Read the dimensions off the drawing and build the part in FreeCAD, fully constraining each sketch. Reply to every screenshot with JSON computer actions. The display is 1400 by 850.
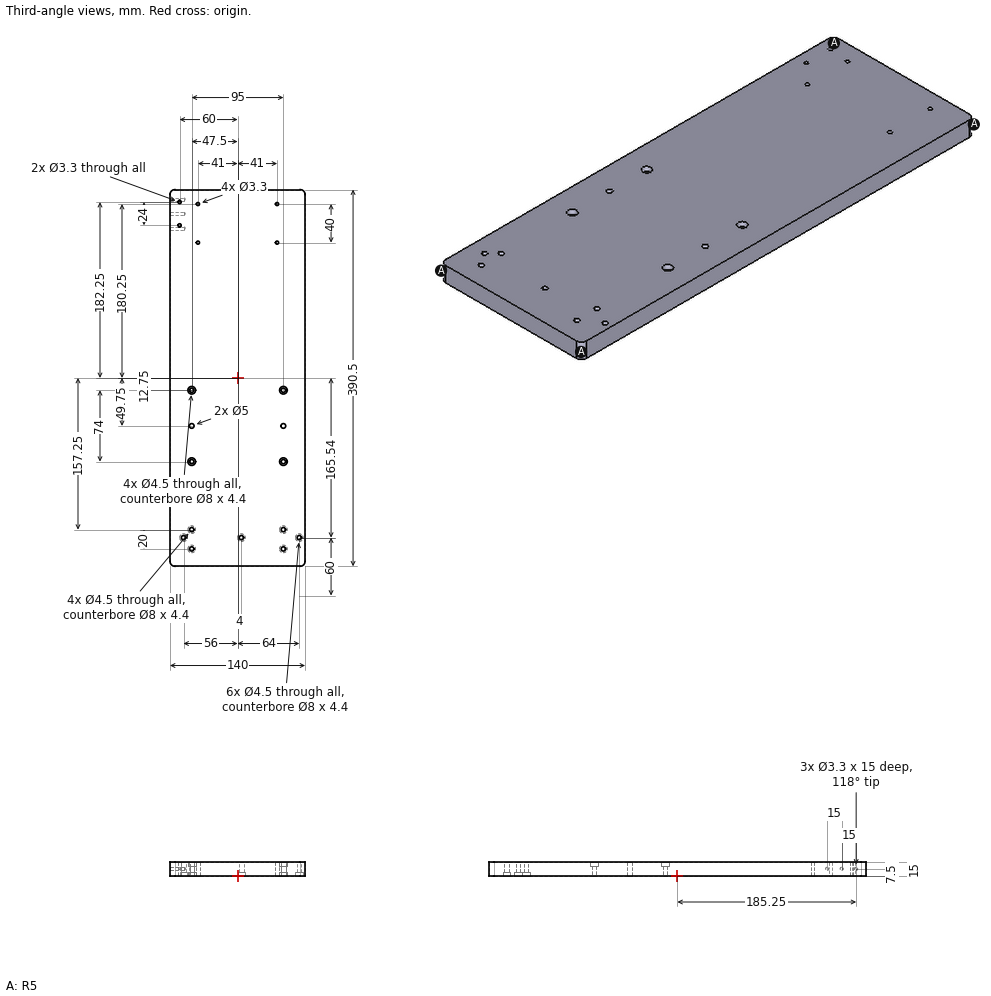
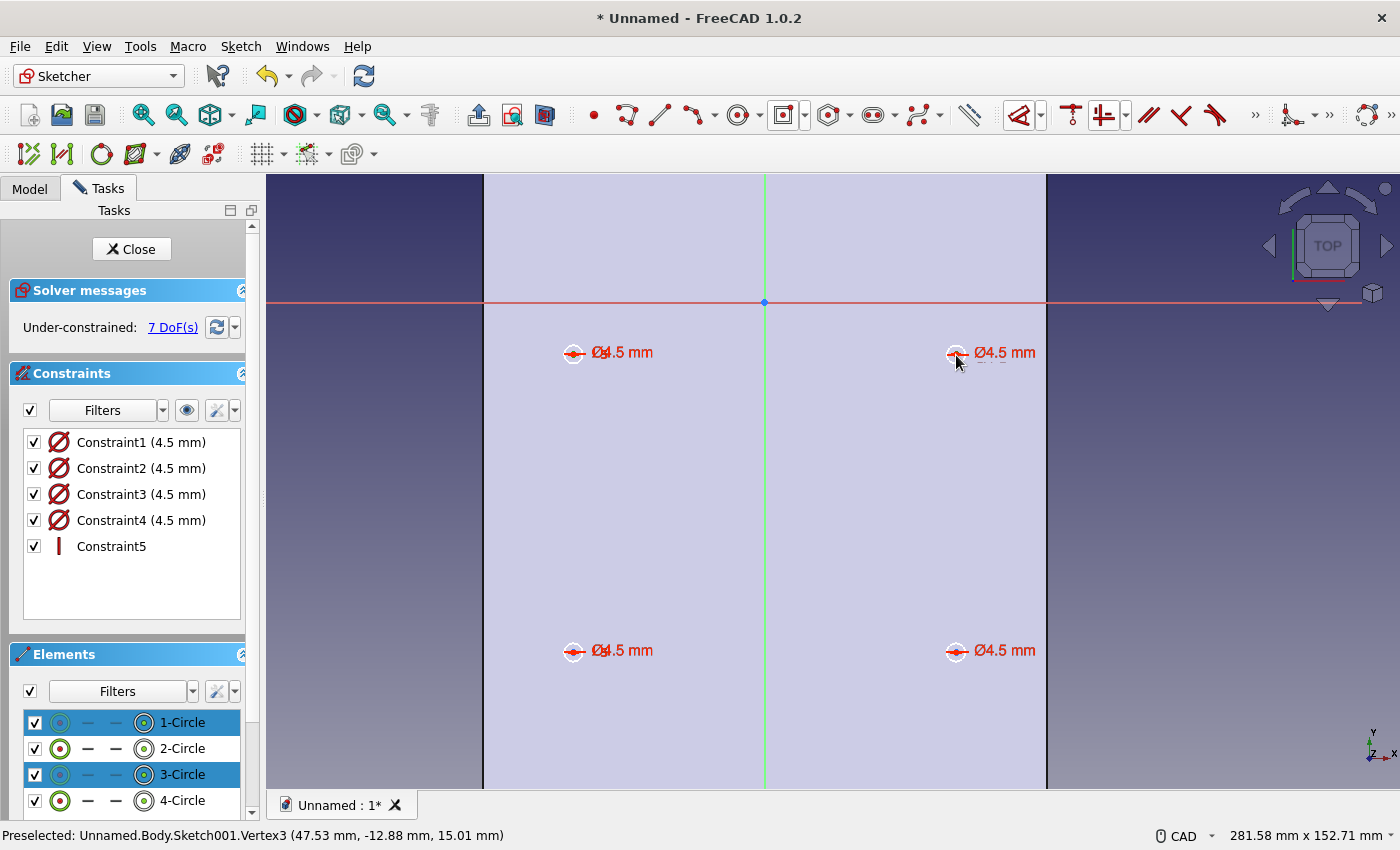
{"action": "key", "text": "h"}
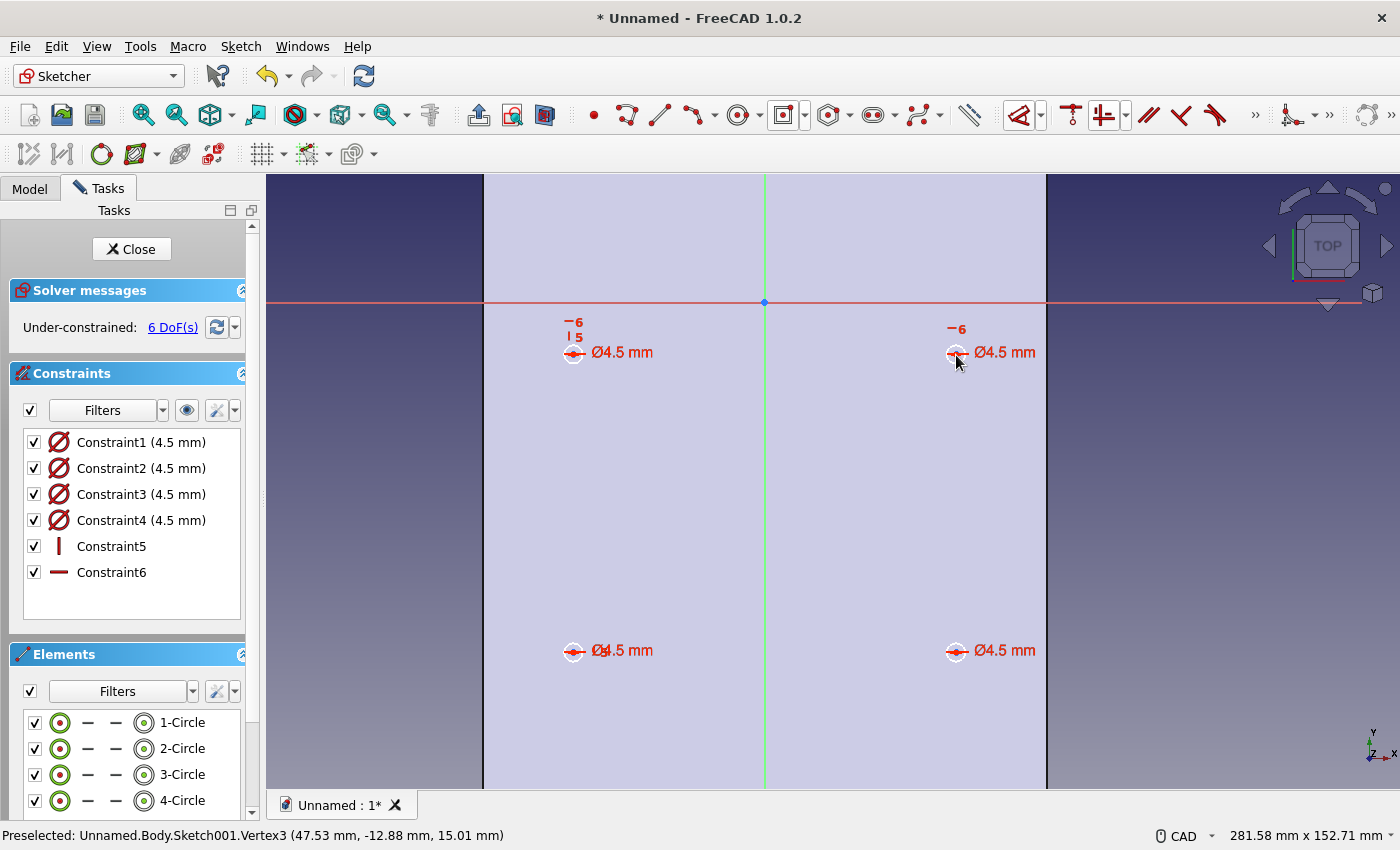
{"action": "left_click", "coordinate": [956, 354]}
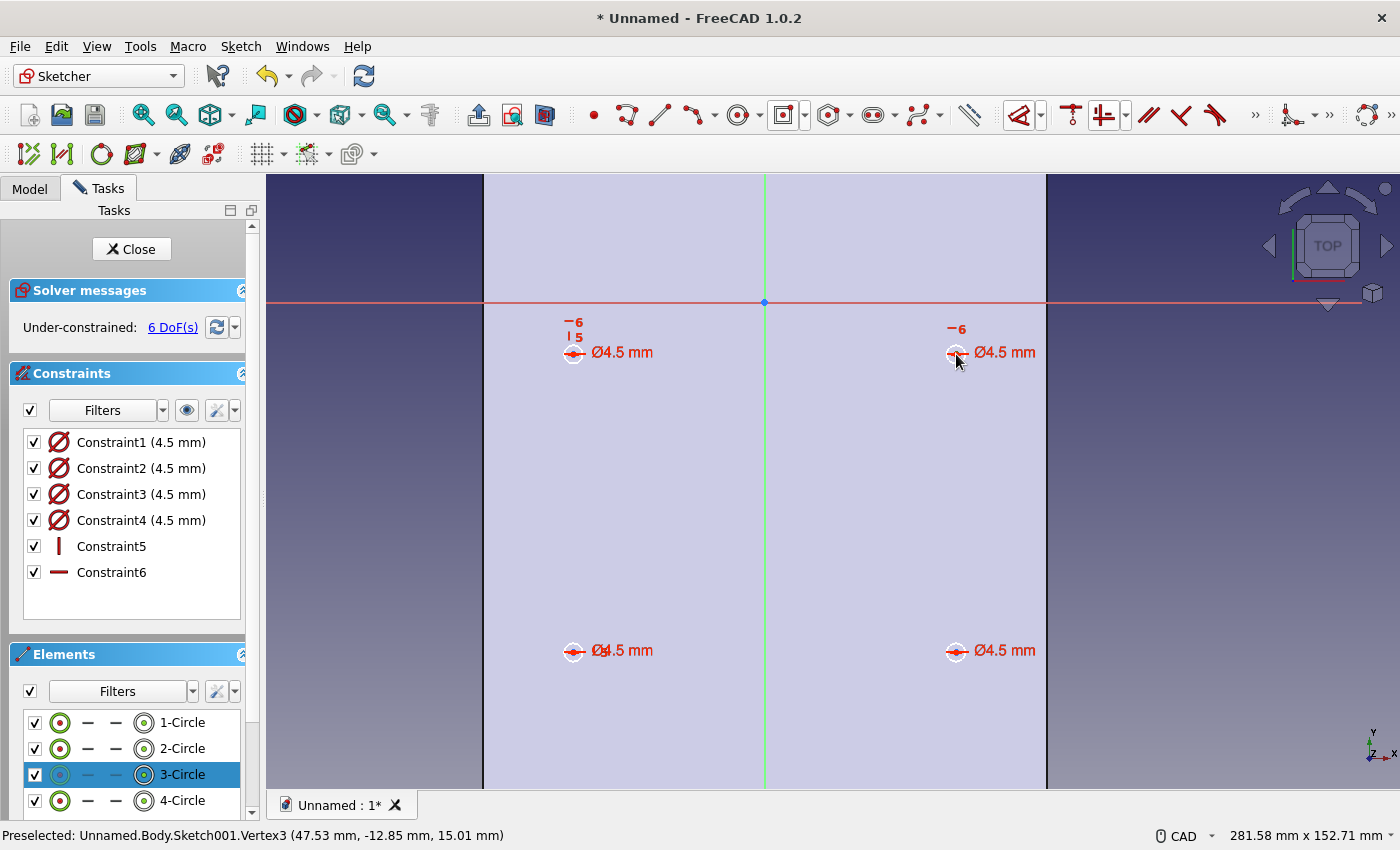
{"action": "left_click", "coordinate": [956, 652]}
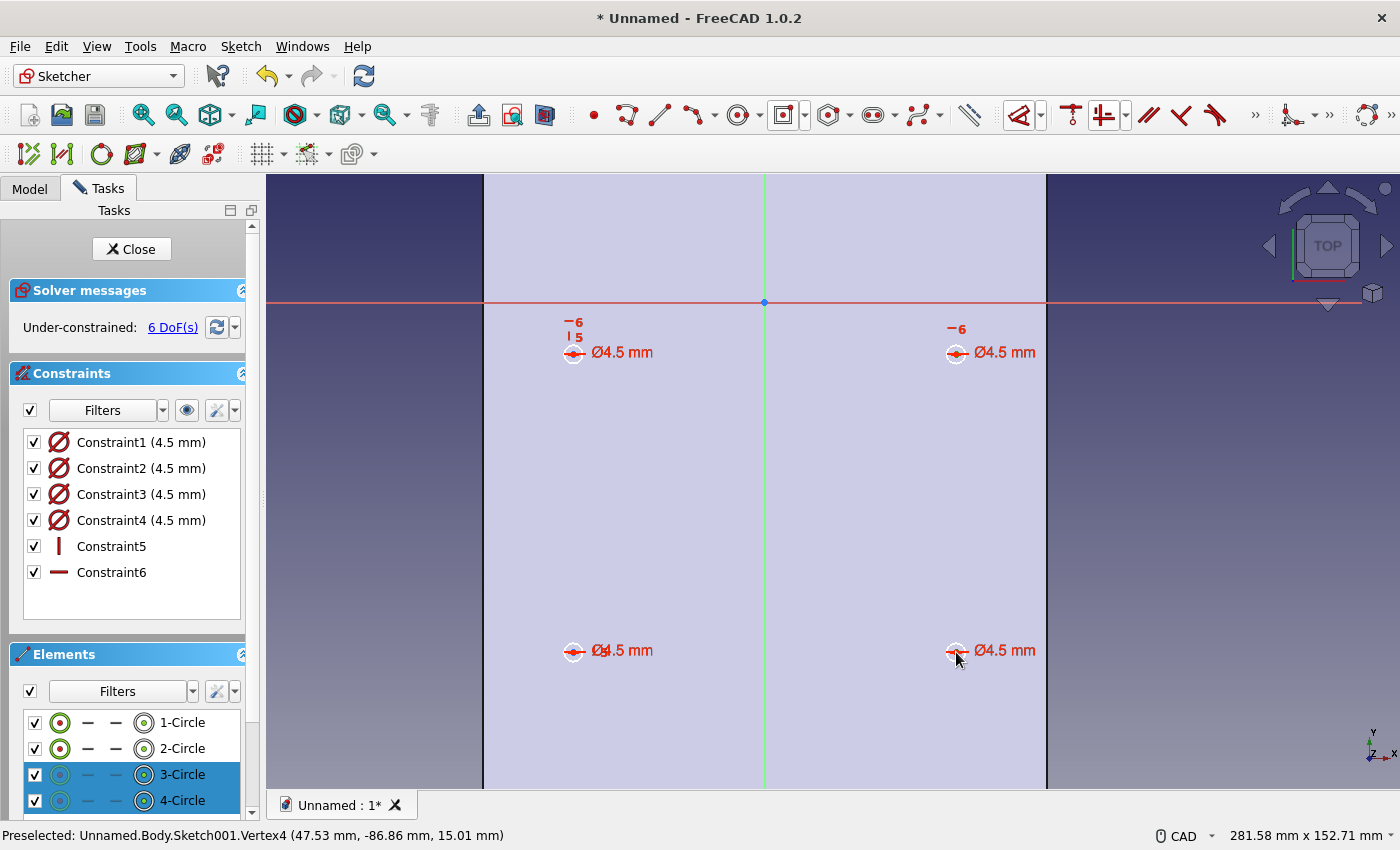
{"action": "left_click", "coordinate": [1126, 116]}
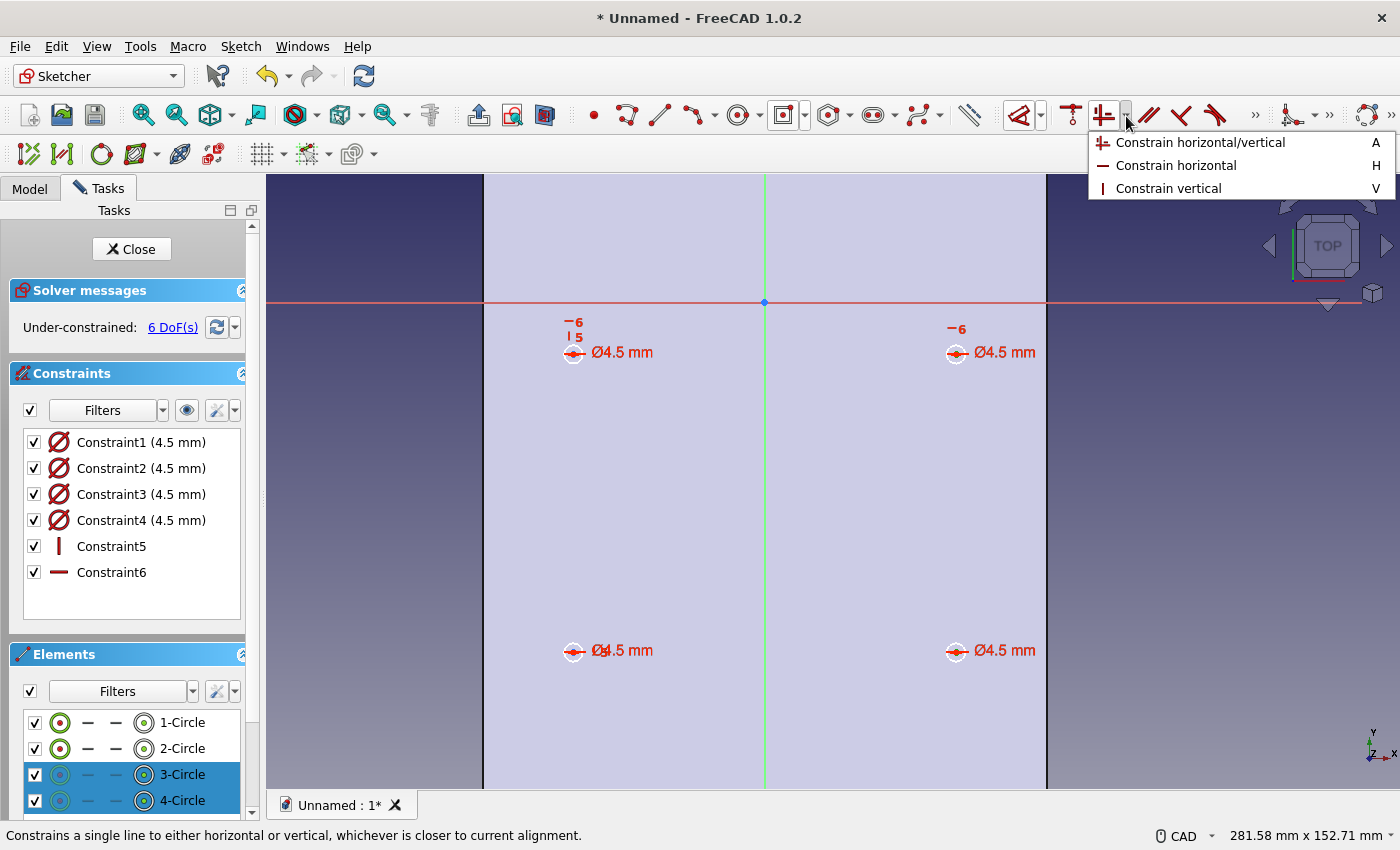
{"action": "left_click", "coordinate": [1242, 188]}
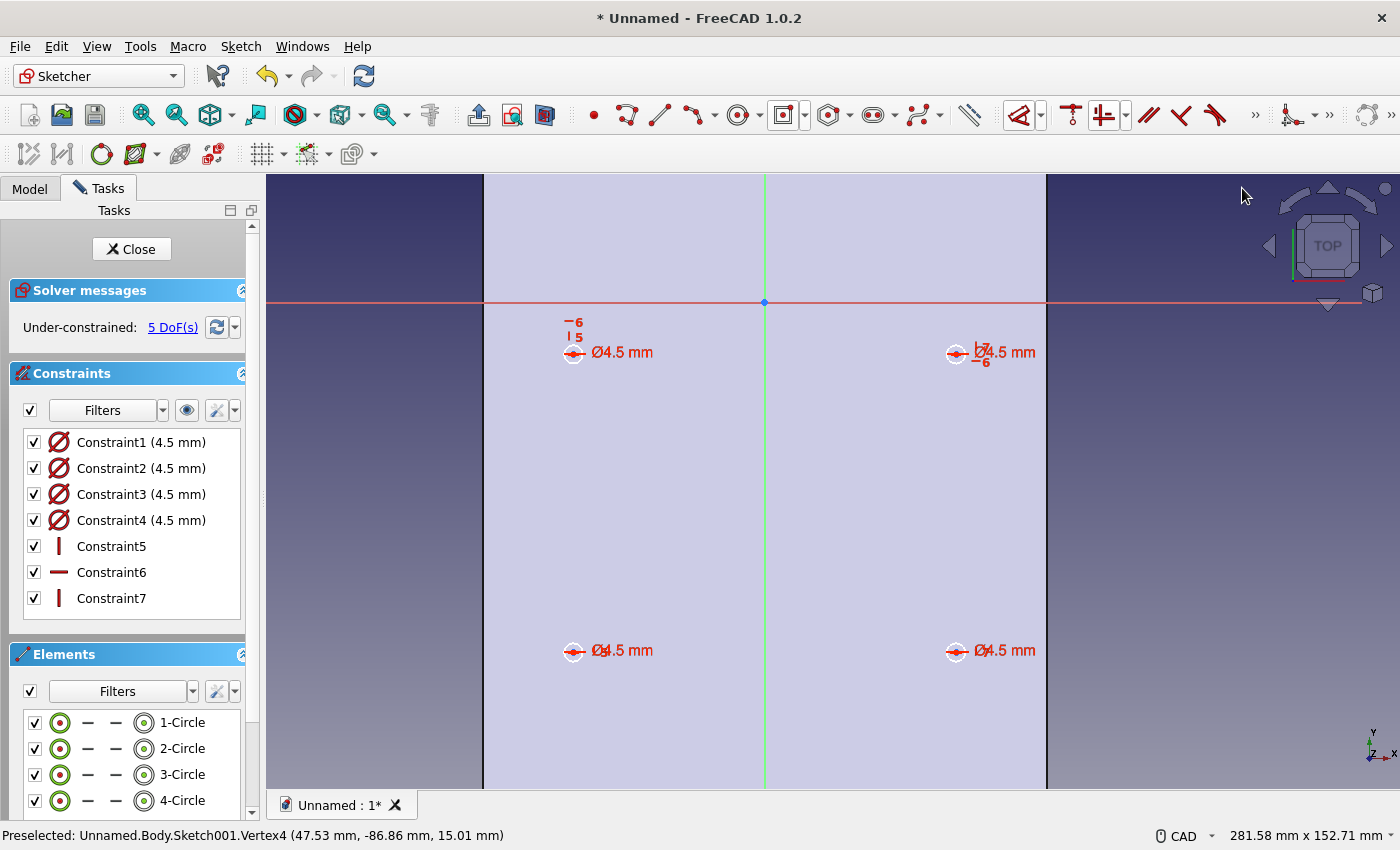
{"action": "left_click", "coordinate": [573, 652]}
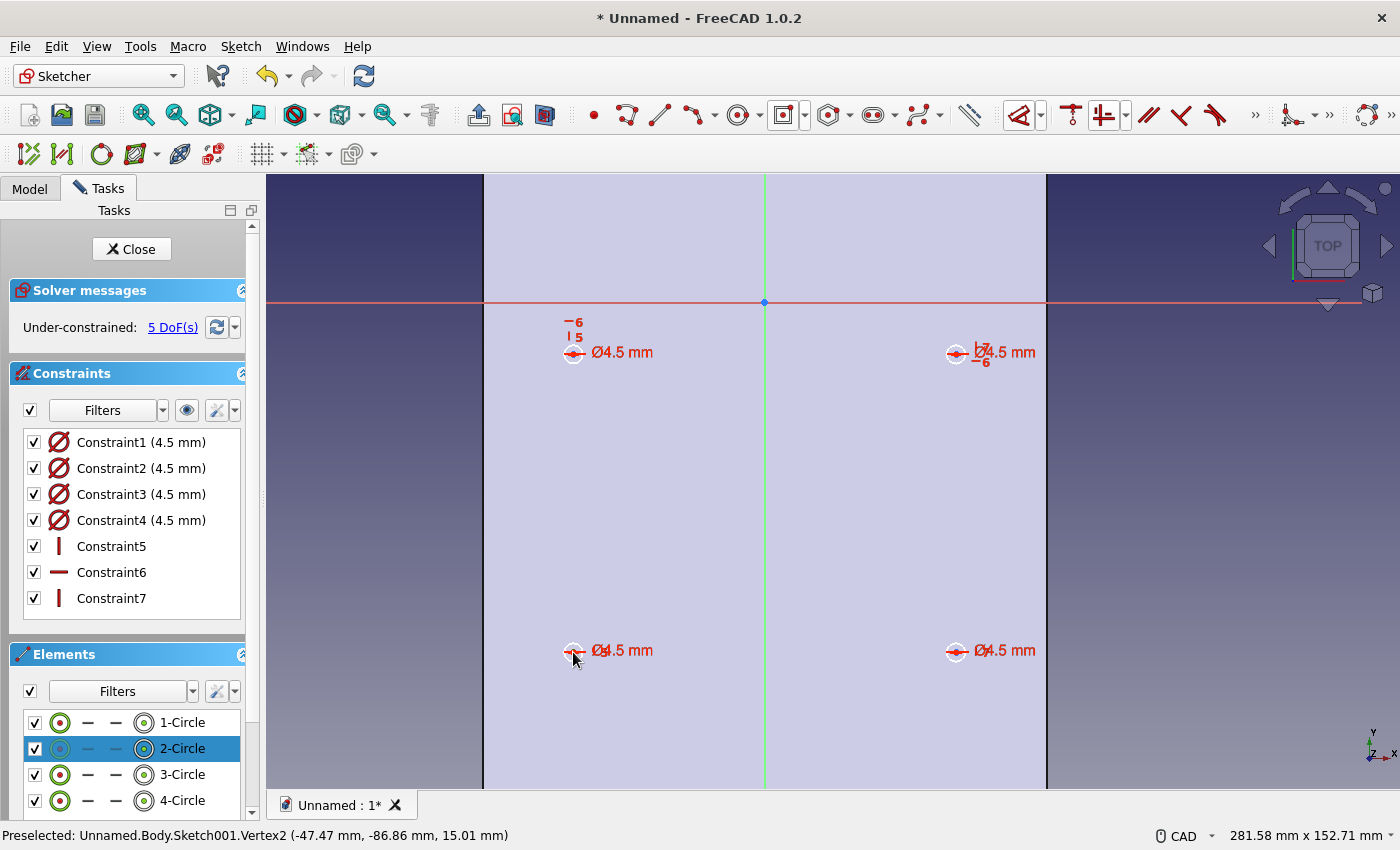
{"action": "left_click", "coordinate": [956, 652]}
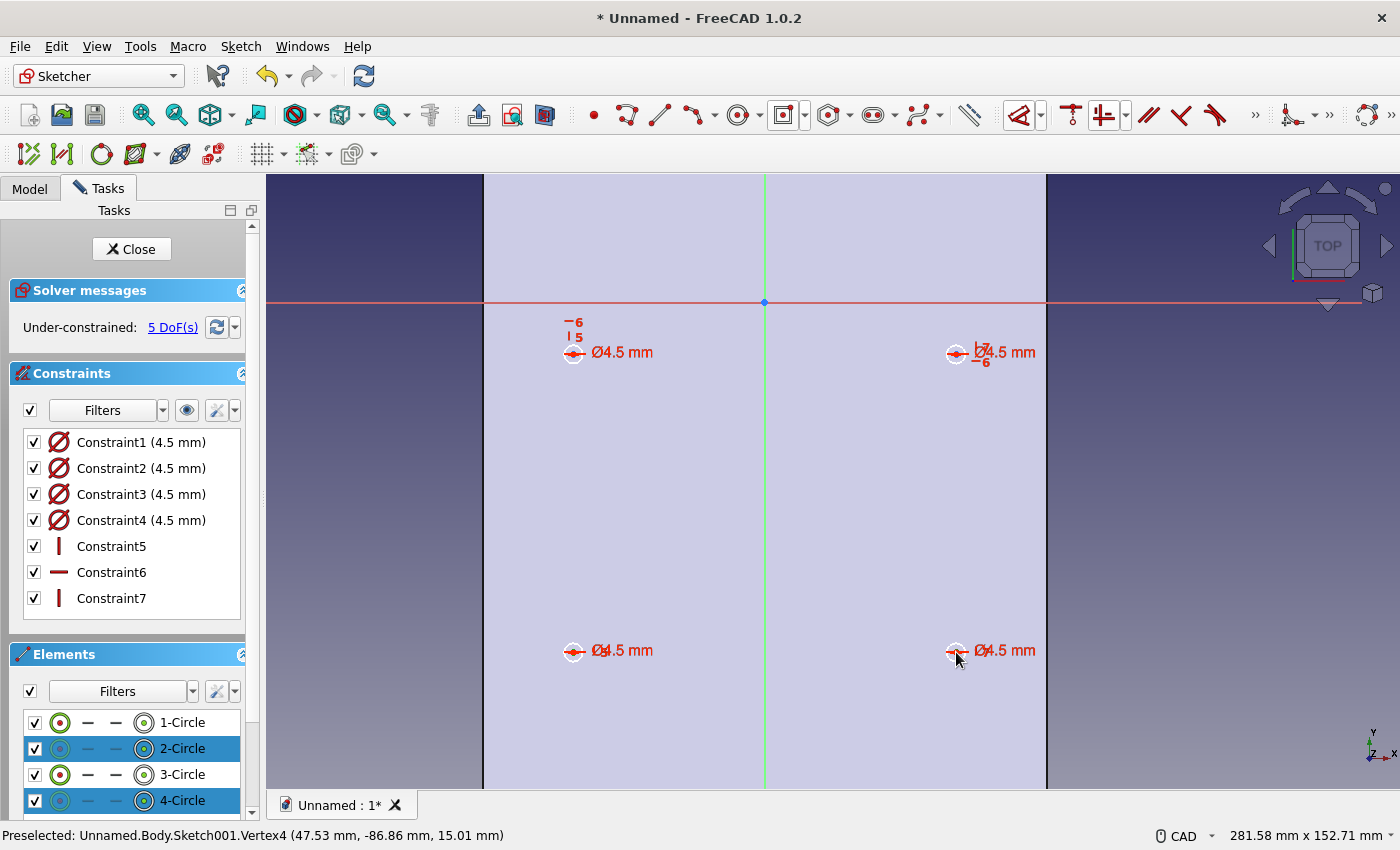
{"action": "left_click", "coordinate": [1126, 116]}